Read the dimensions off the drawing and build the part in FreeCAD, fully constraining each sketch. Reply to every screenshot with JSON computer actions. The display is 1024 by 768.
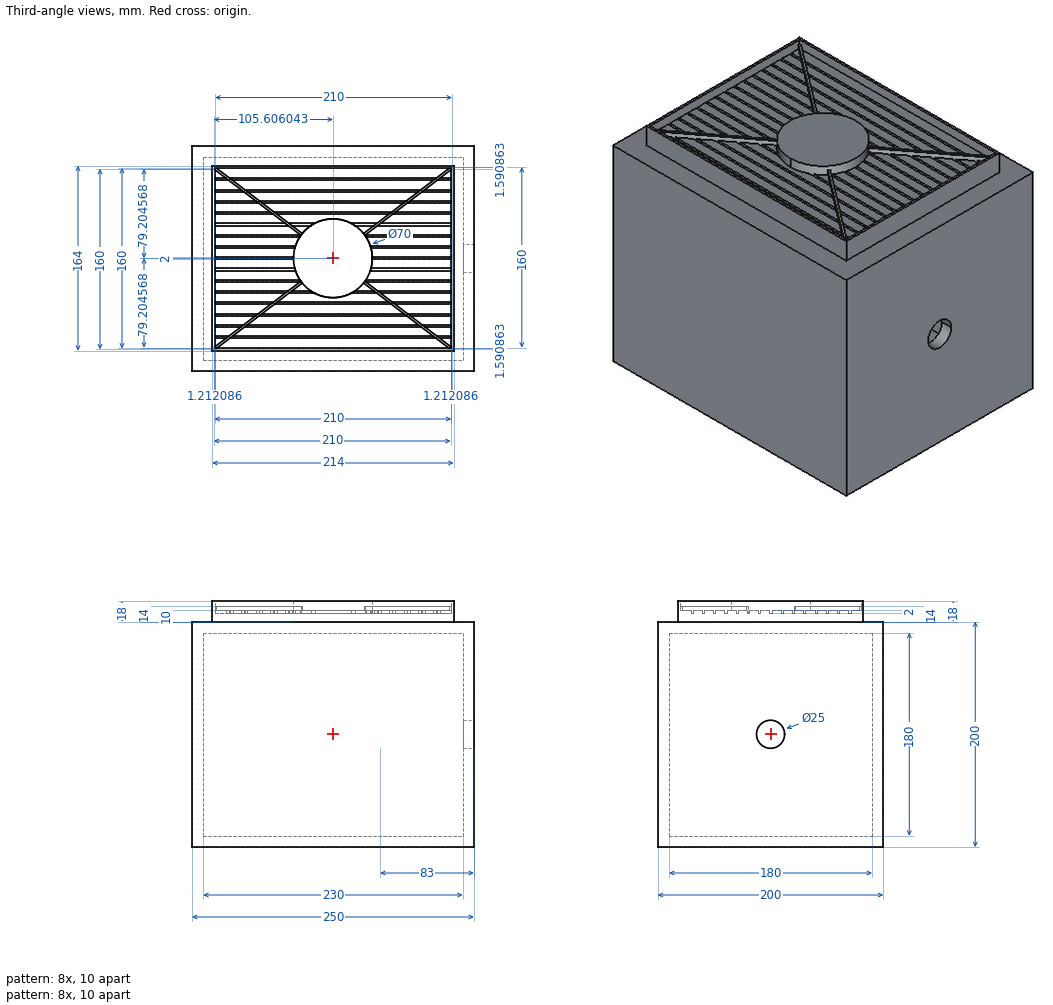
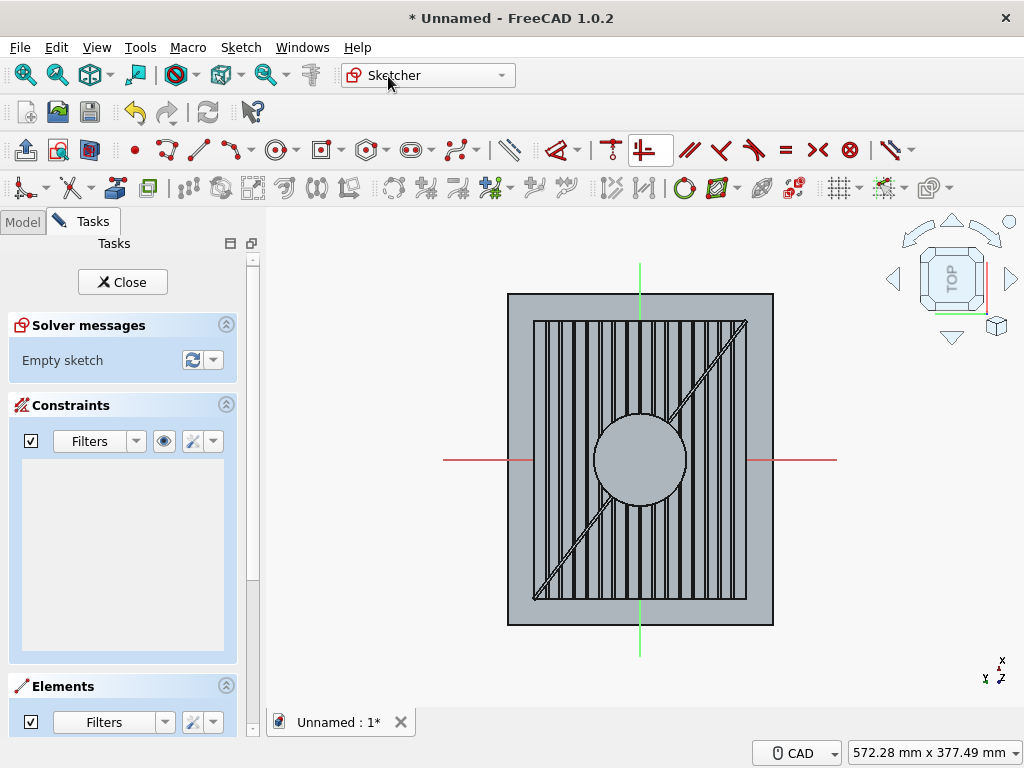
{"action": "left_click", "coordinate": [90, 150]}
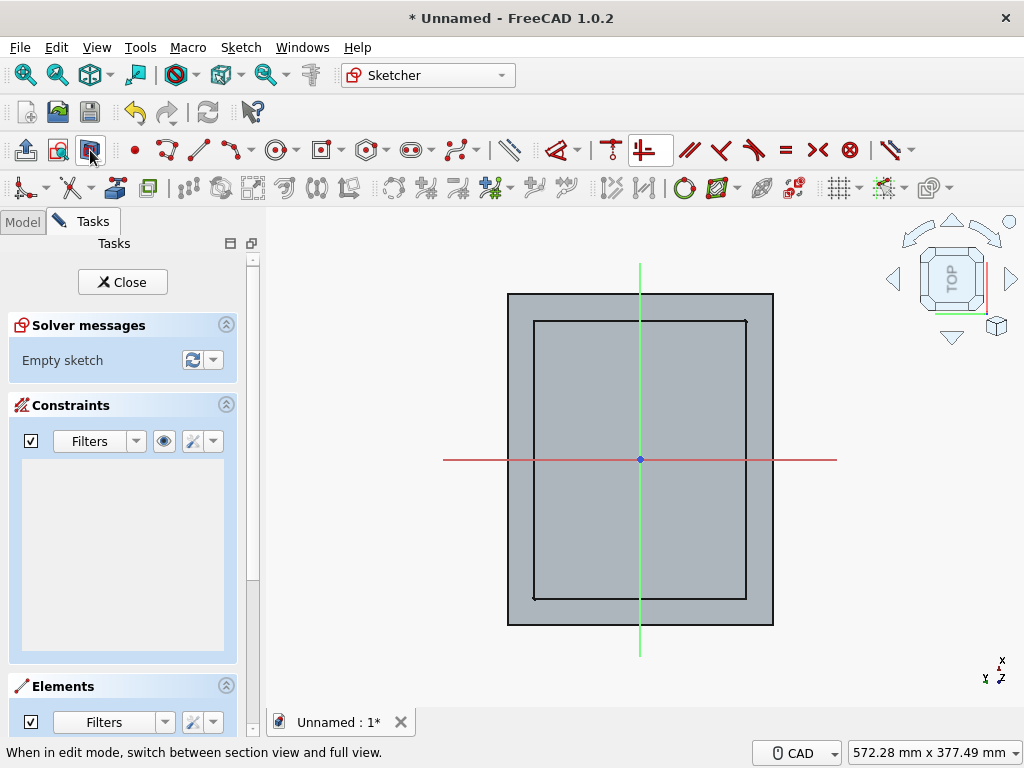
{"action": "left_click", "coordinate": [168, 150]}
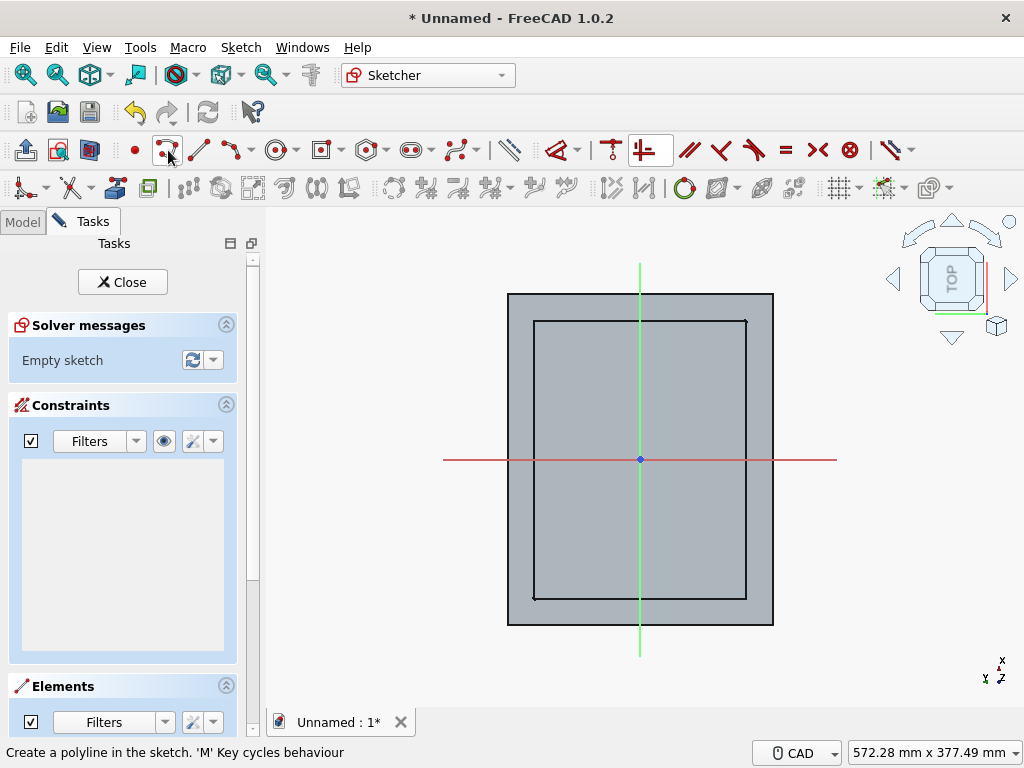
{"action": "left_click", "coordinate": [745, 600]}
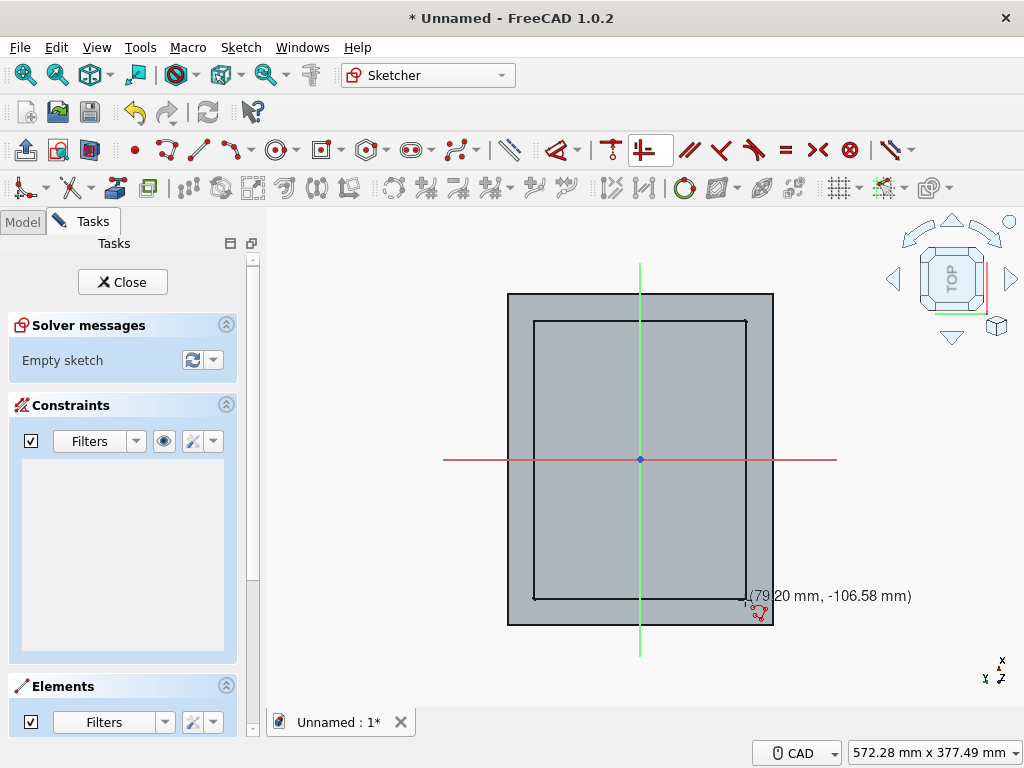
{"action": "scroll", "coordinate": [747, 598], "scroll_direction": "up", "scroll_amount": 9}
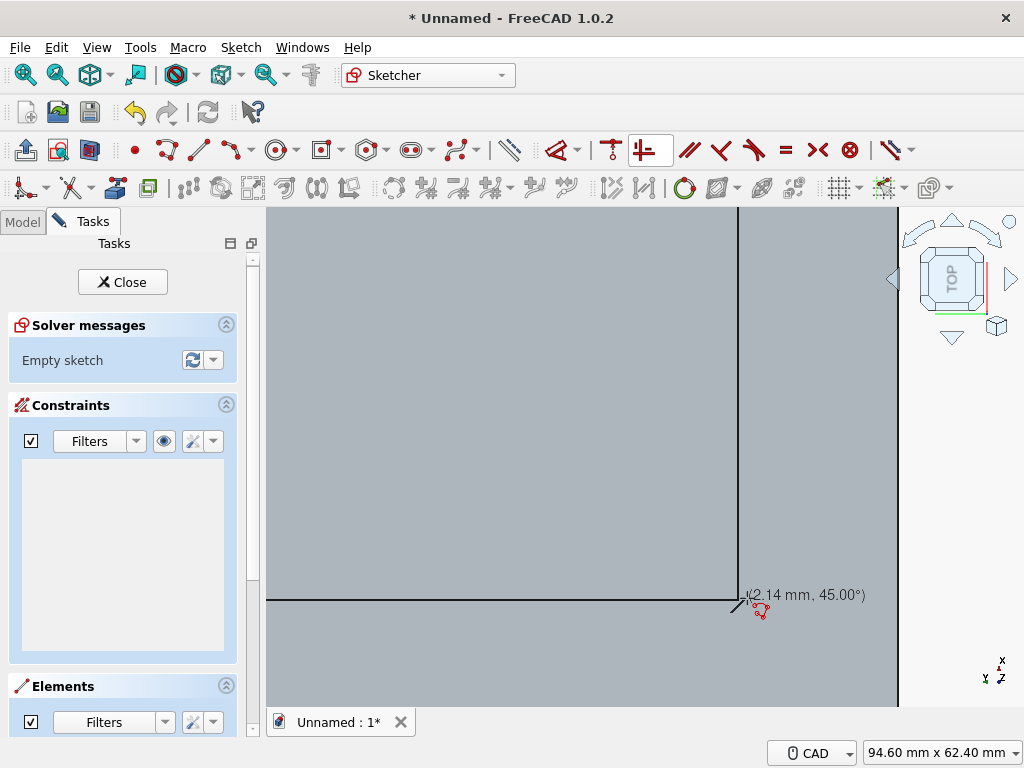
{"action": "left_click", "coordinate": [744, 595]}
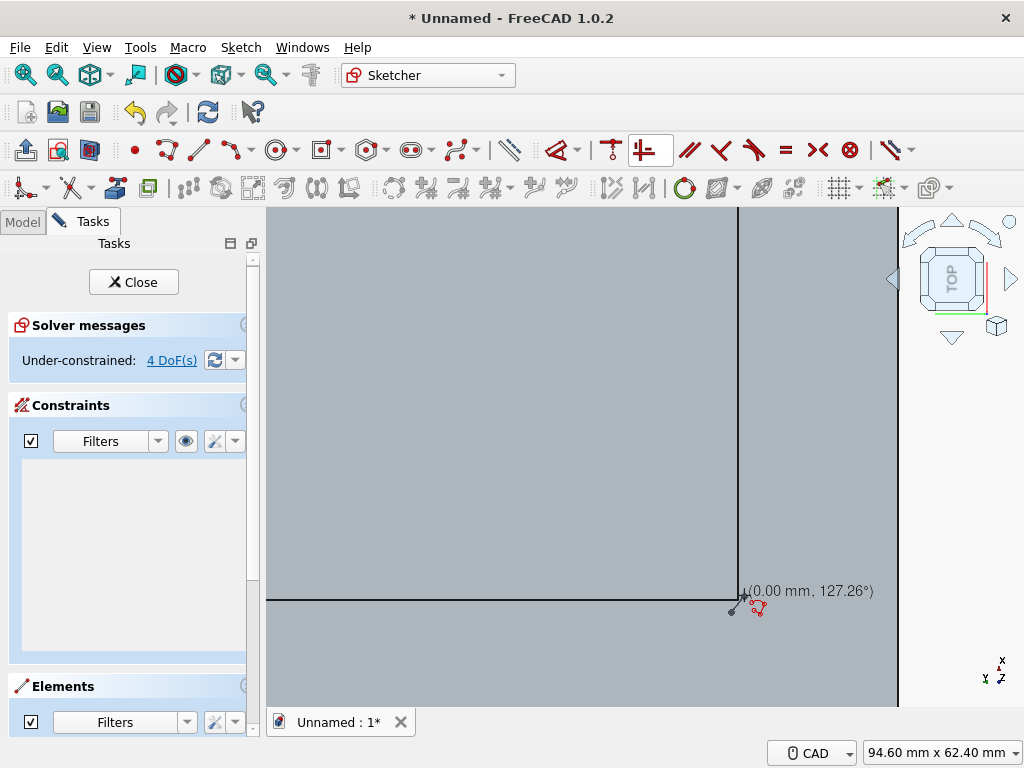
{"action": "scroll", "coordinate": [698, 634], "scroll_direction": "down", "scroll_amount": 8}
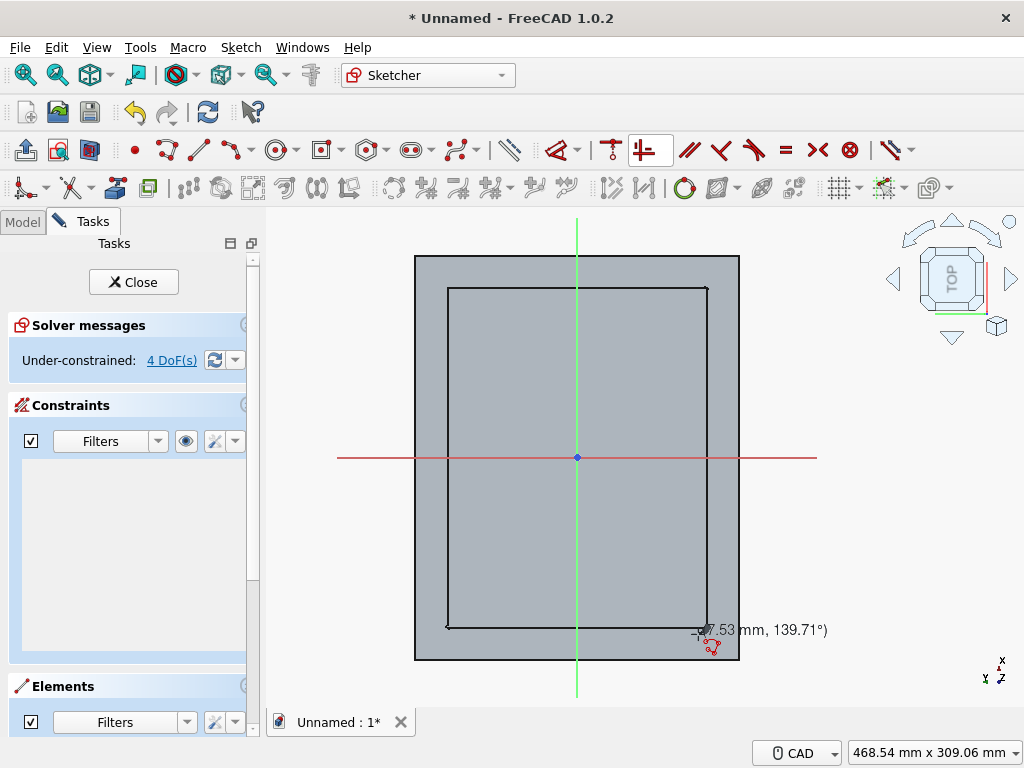
{"action": "left_click", "coordinate": [449, 287]}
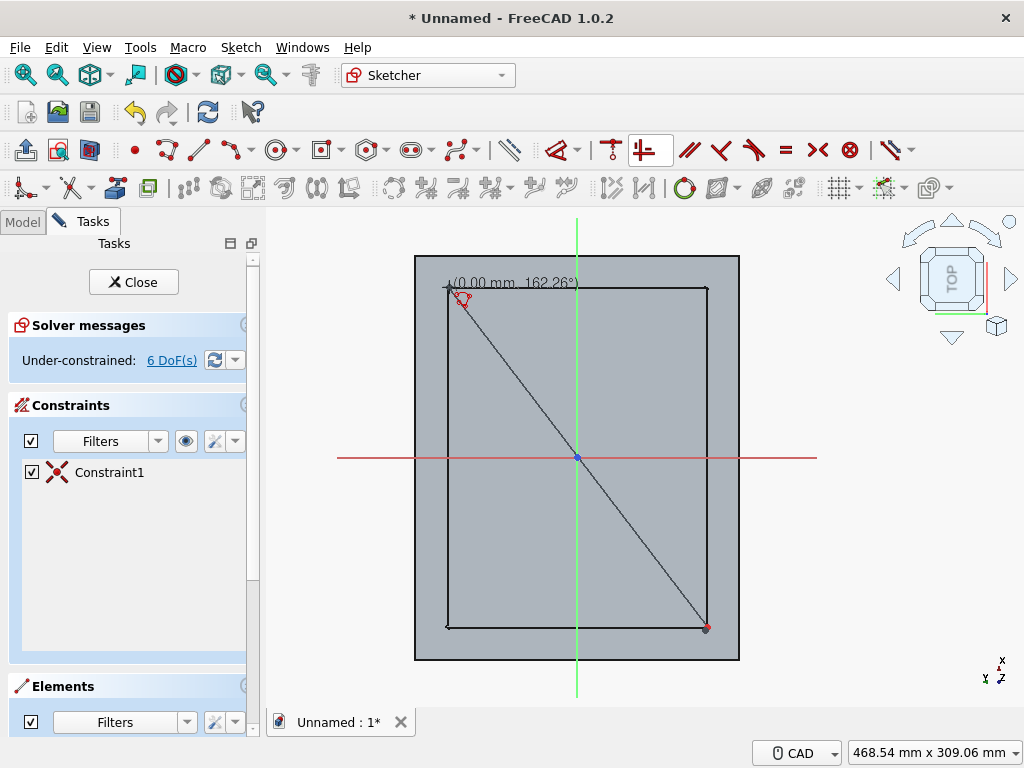
{"action": "scroll", "coordinate": [446, 289], "scroll_direction": "up", "scroll_amount": 8}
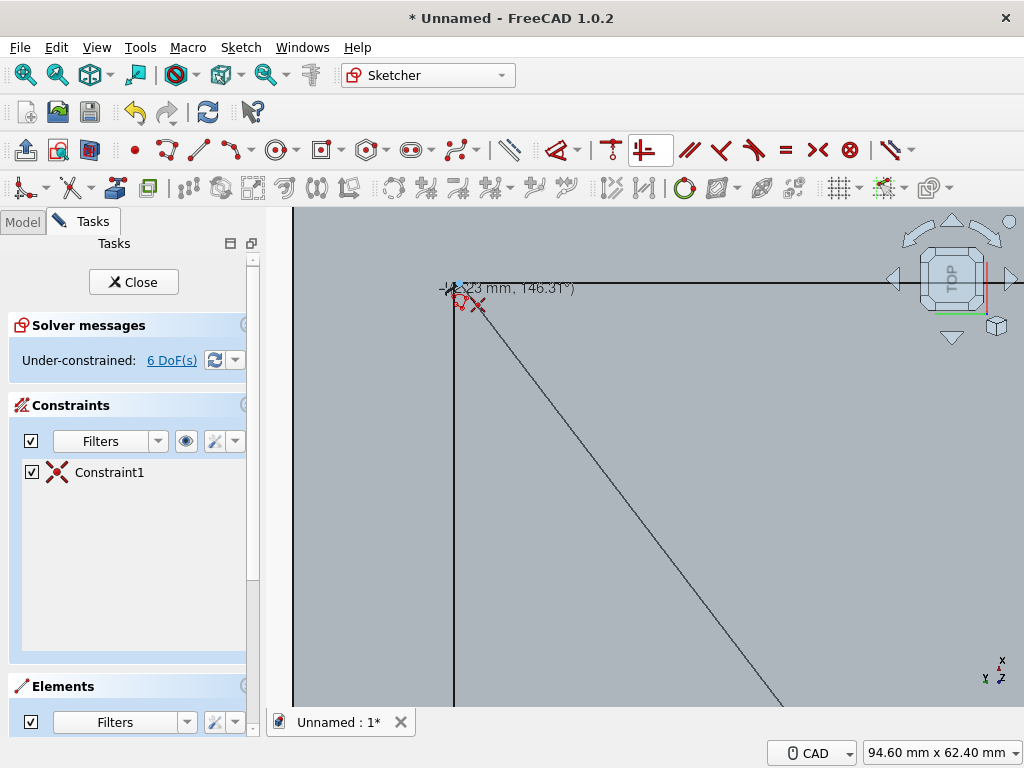
{"action": "left_click", "coordinate": [447, 288]}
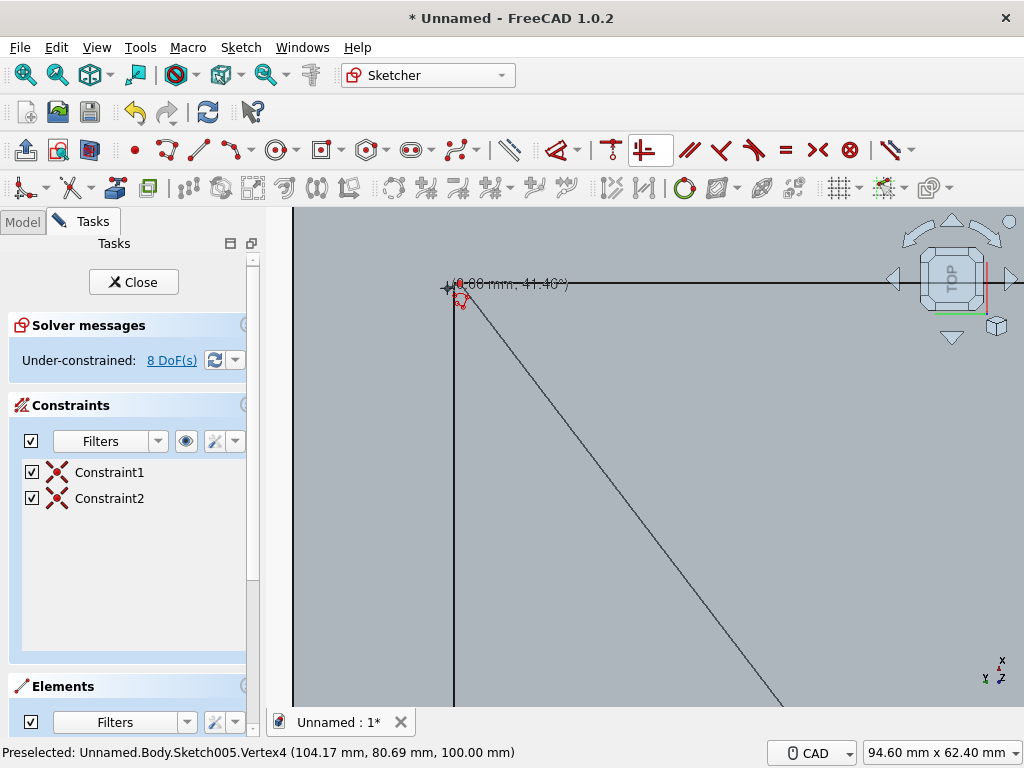
{"action": "scroll", "coordinate": [445, 288], "scroll_direction": "down", "scroll_amount": 8}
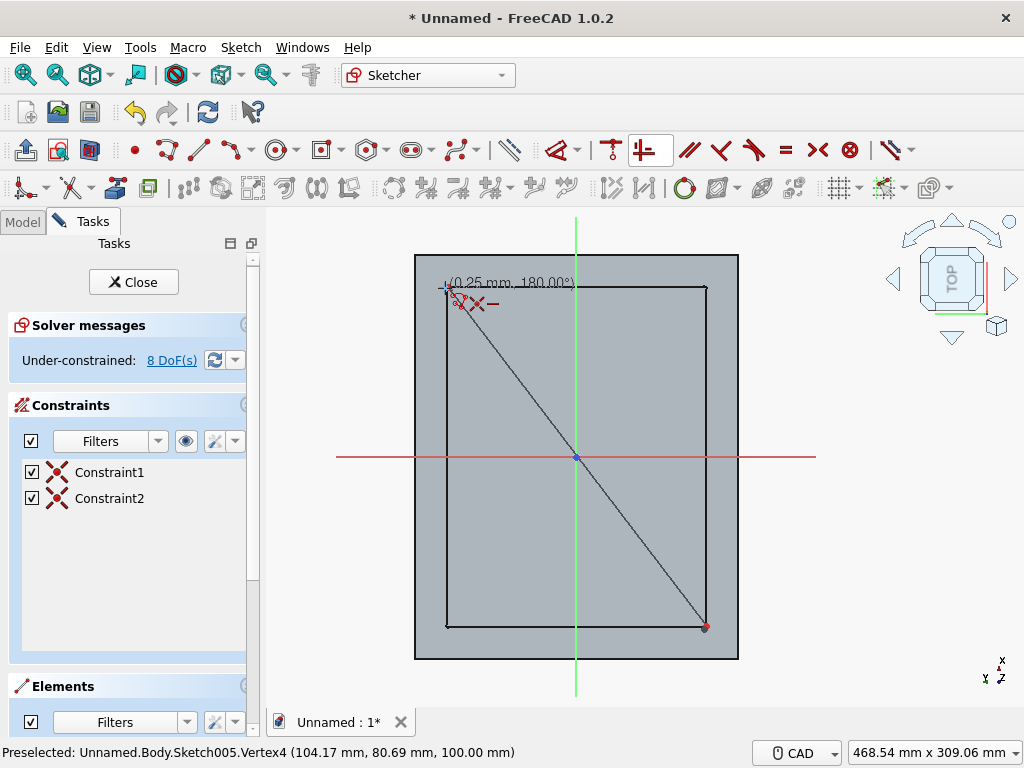
{"action": "scroll", "coordinate": [704, 628], "scroll_direction": "up", "scroll_amount": 12}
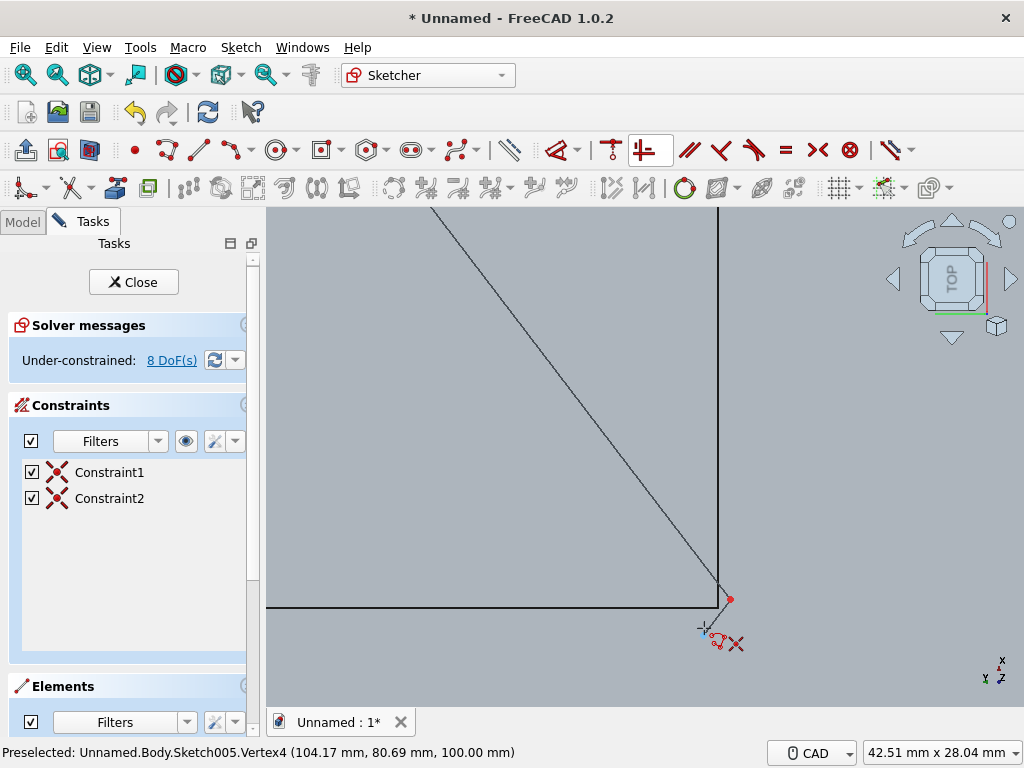
{"action": "left_click", "coordinate": [703, 622]}
{"action": "key", "text": "Escape"}
{"action": "key", "text": "Escape"}